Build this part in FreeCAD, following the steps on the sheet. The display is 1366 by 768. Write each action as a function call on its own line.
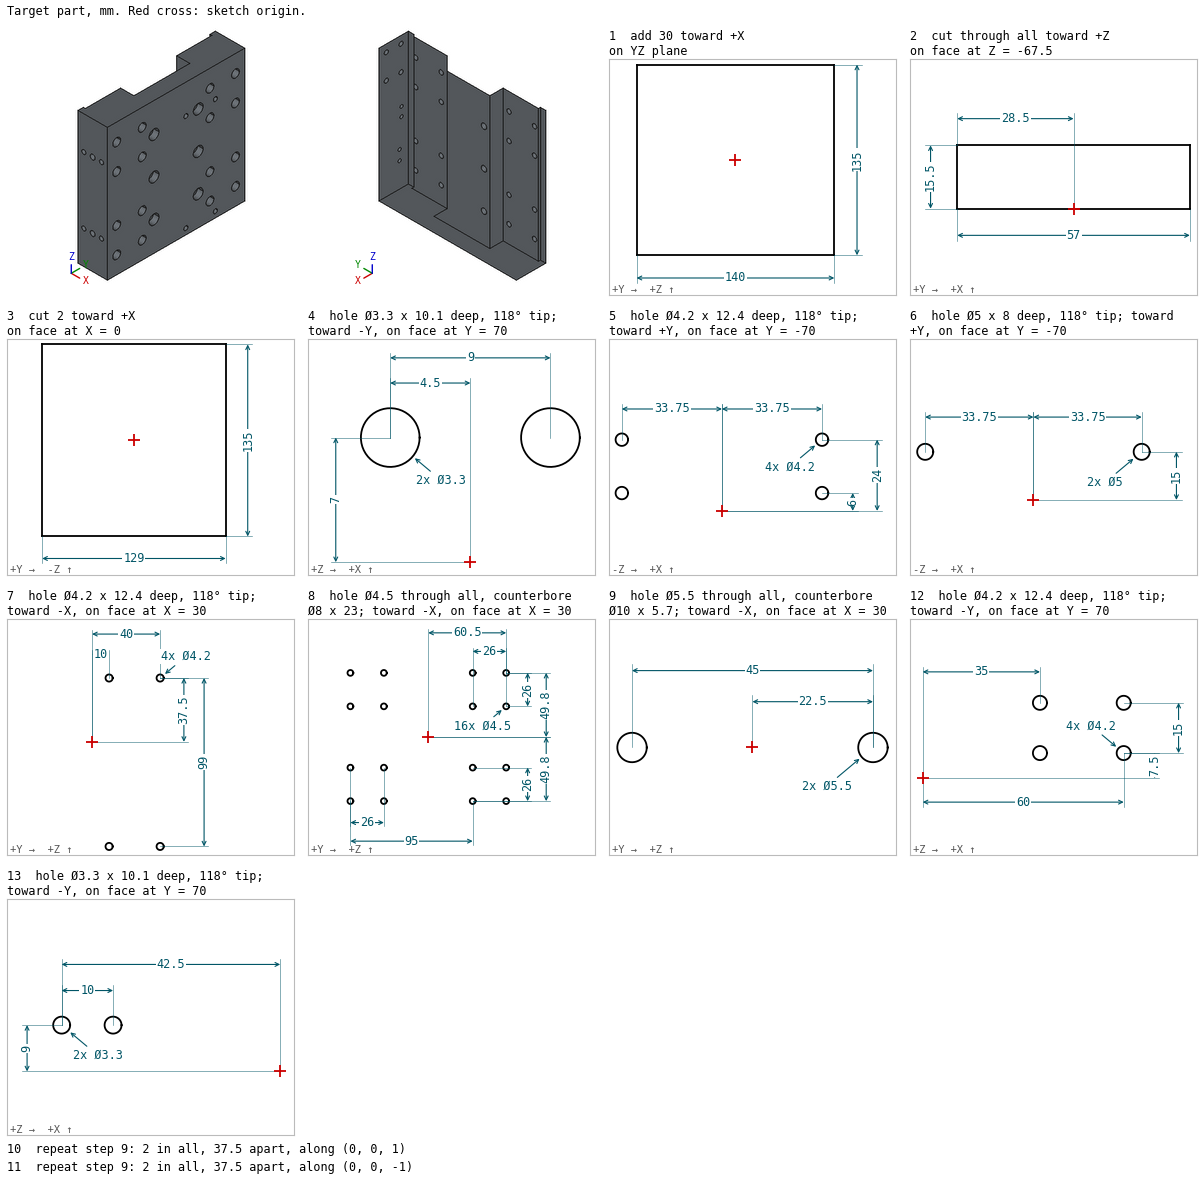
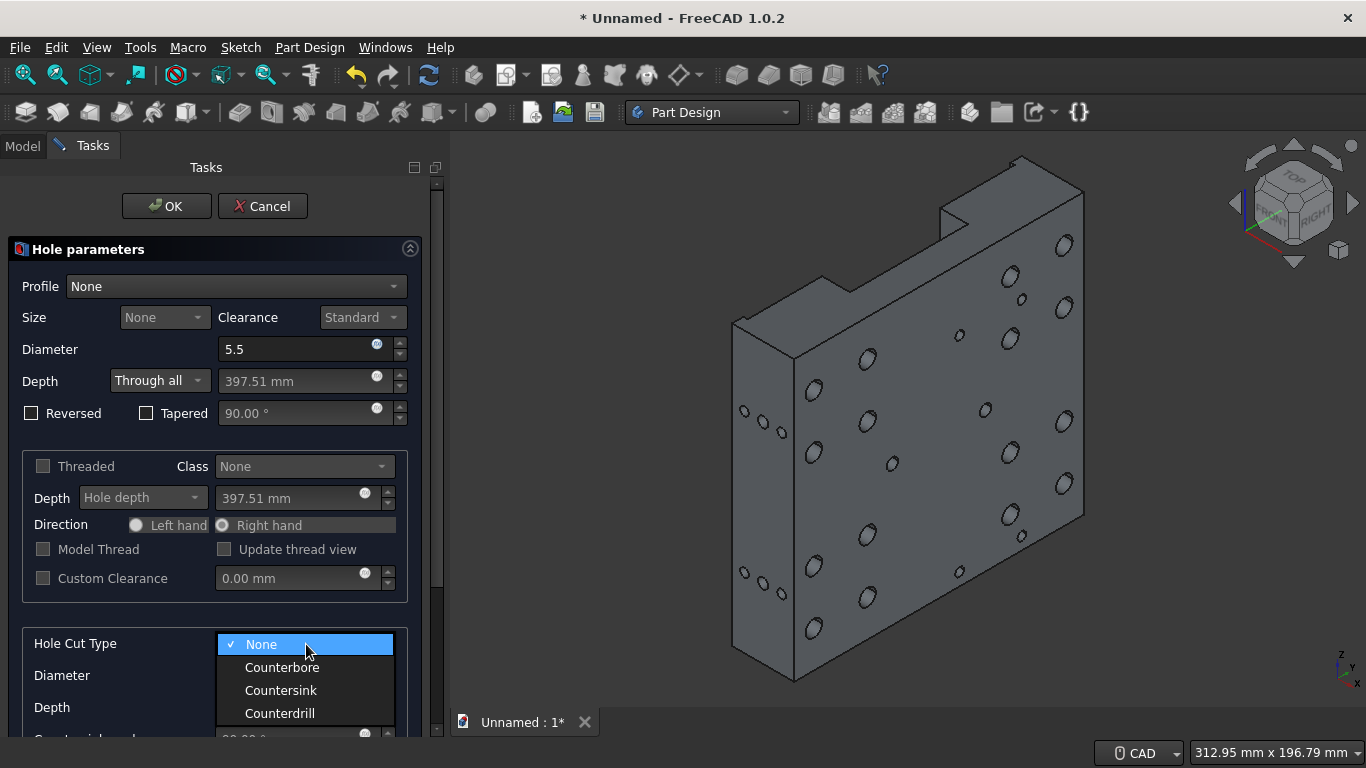
click(304, 668)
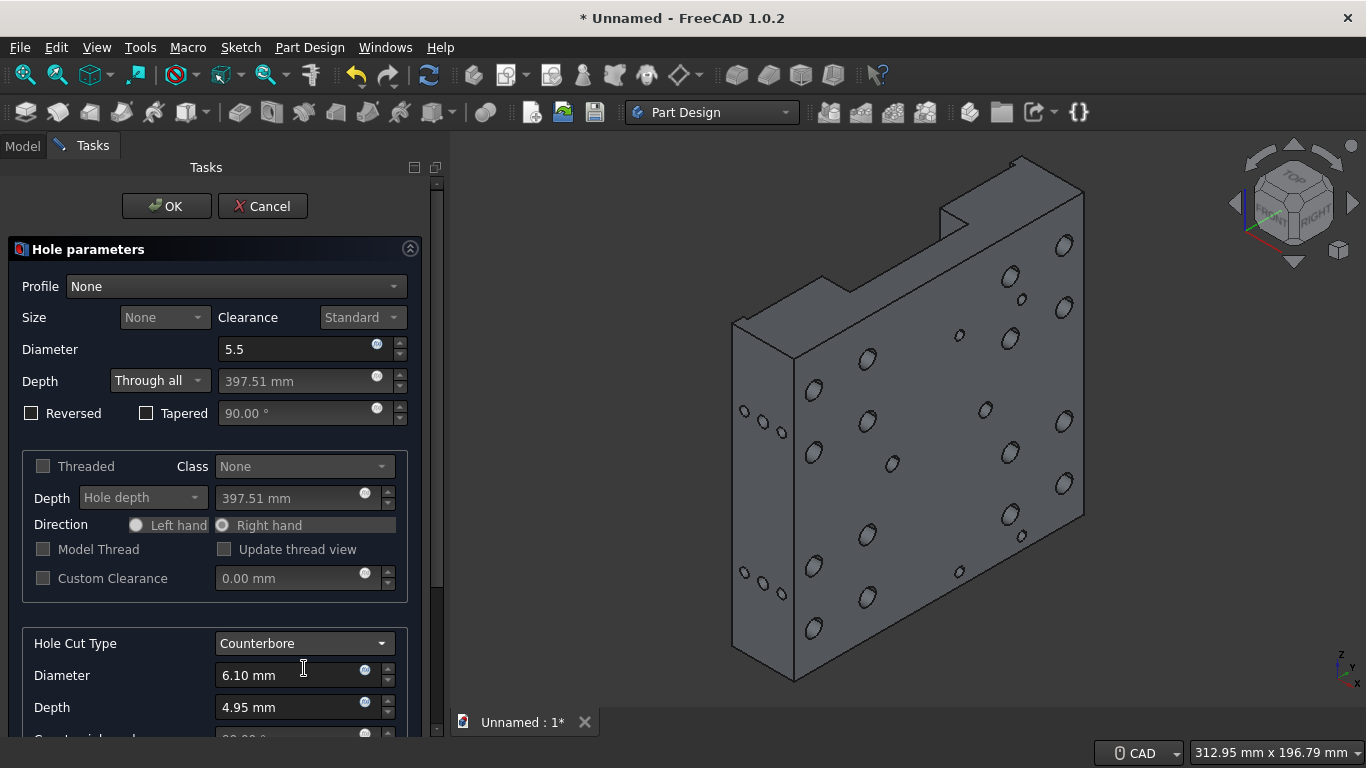
triple_click(298, 675)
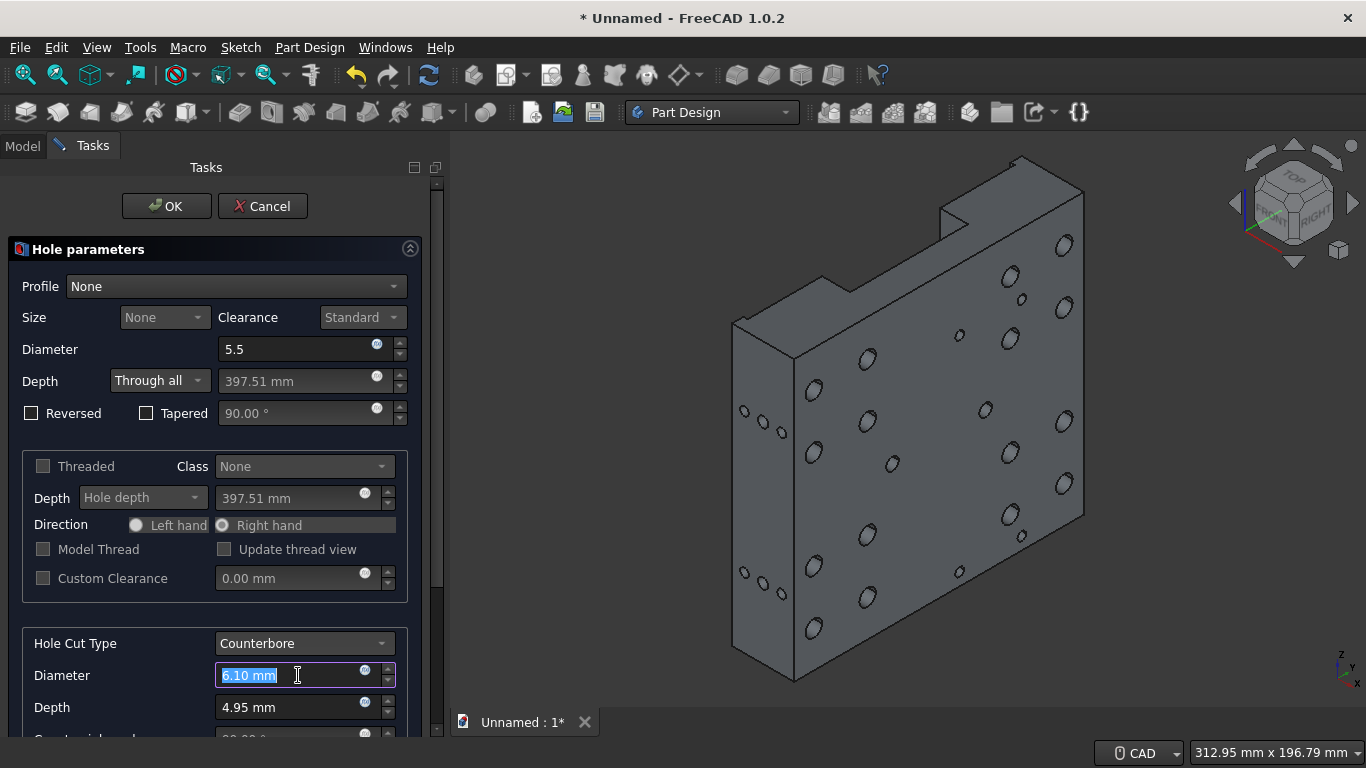
text(10)
key(Tab)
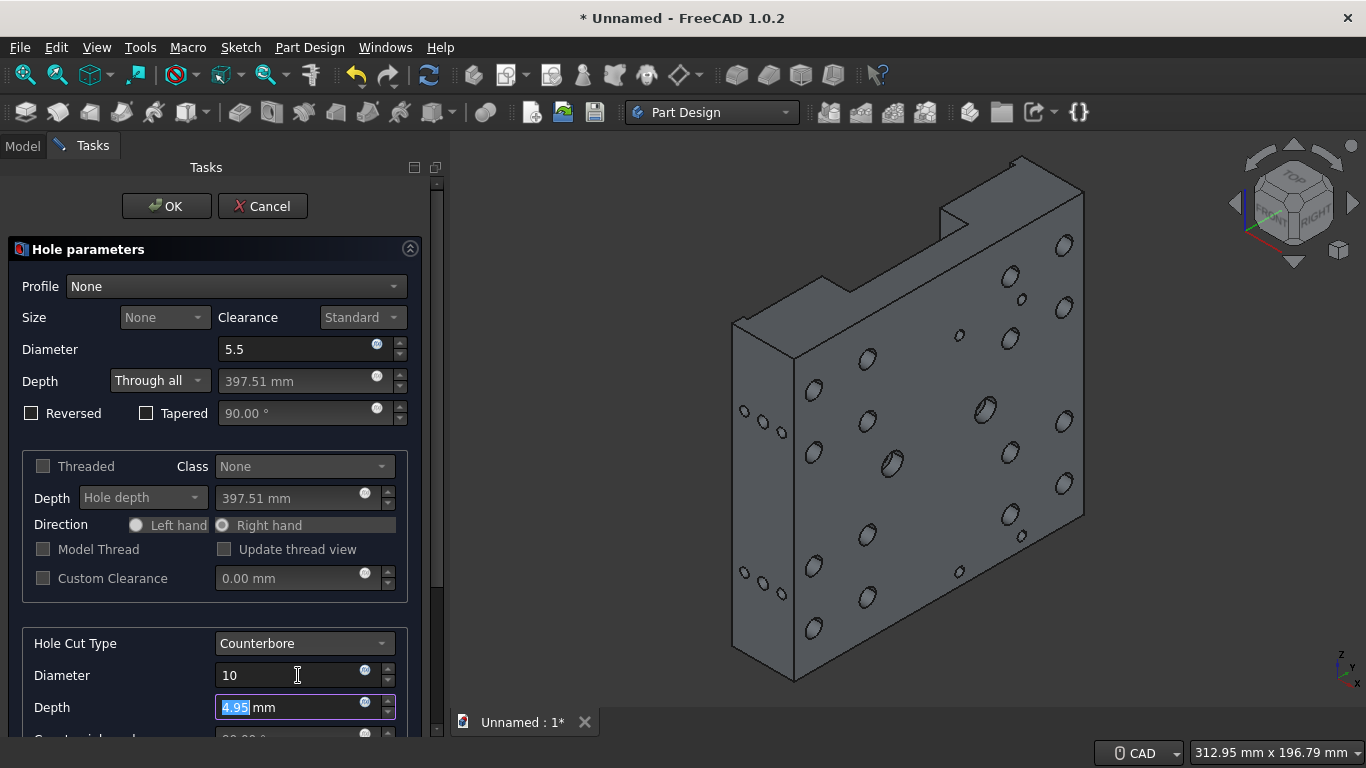
text(5.7)
key(Tab)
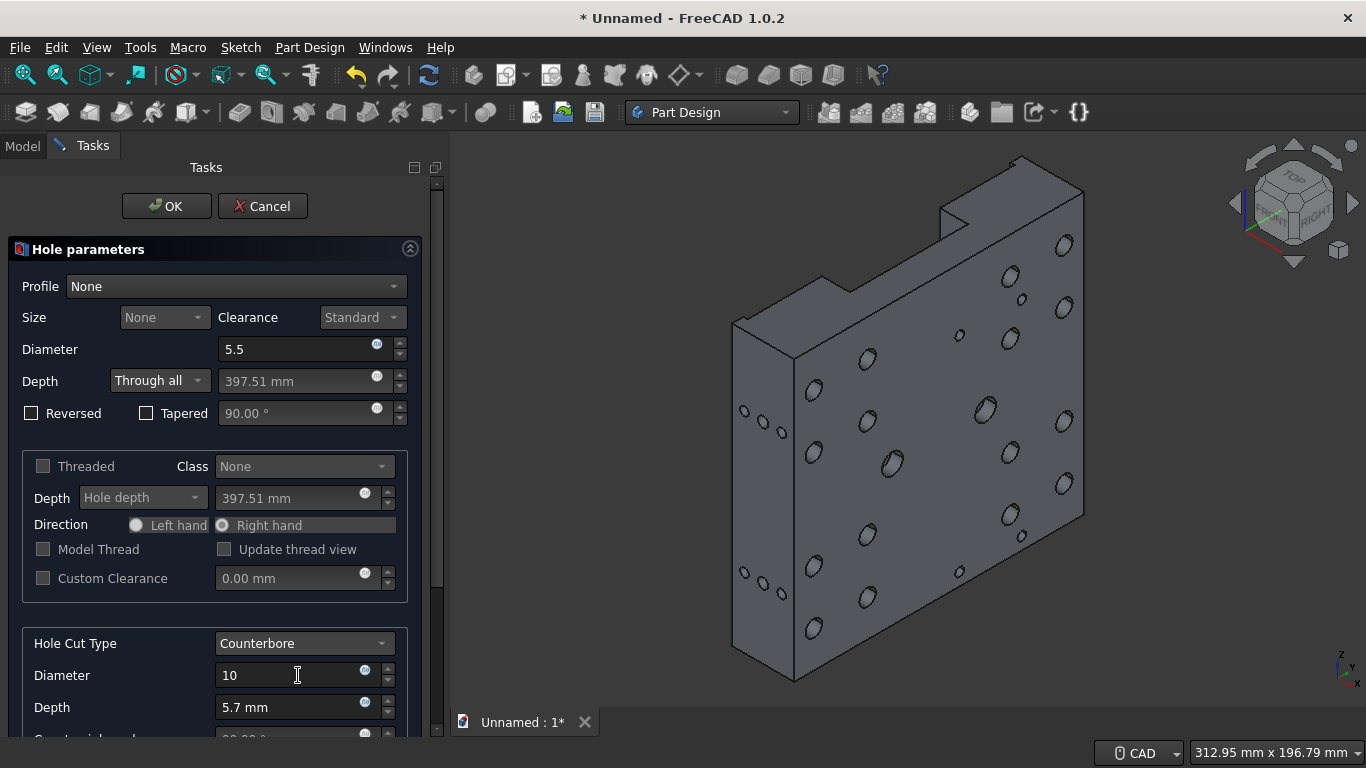
click(167, 206)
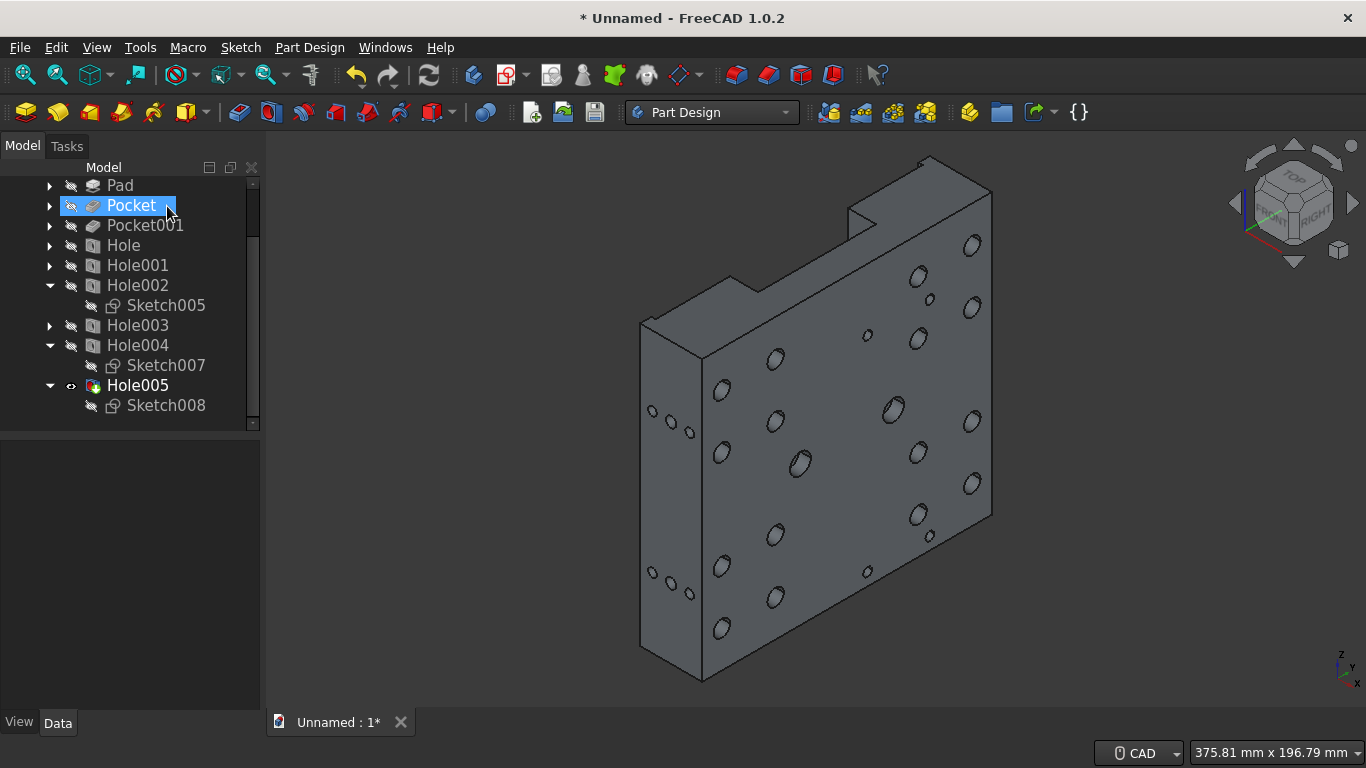
click(116, 386)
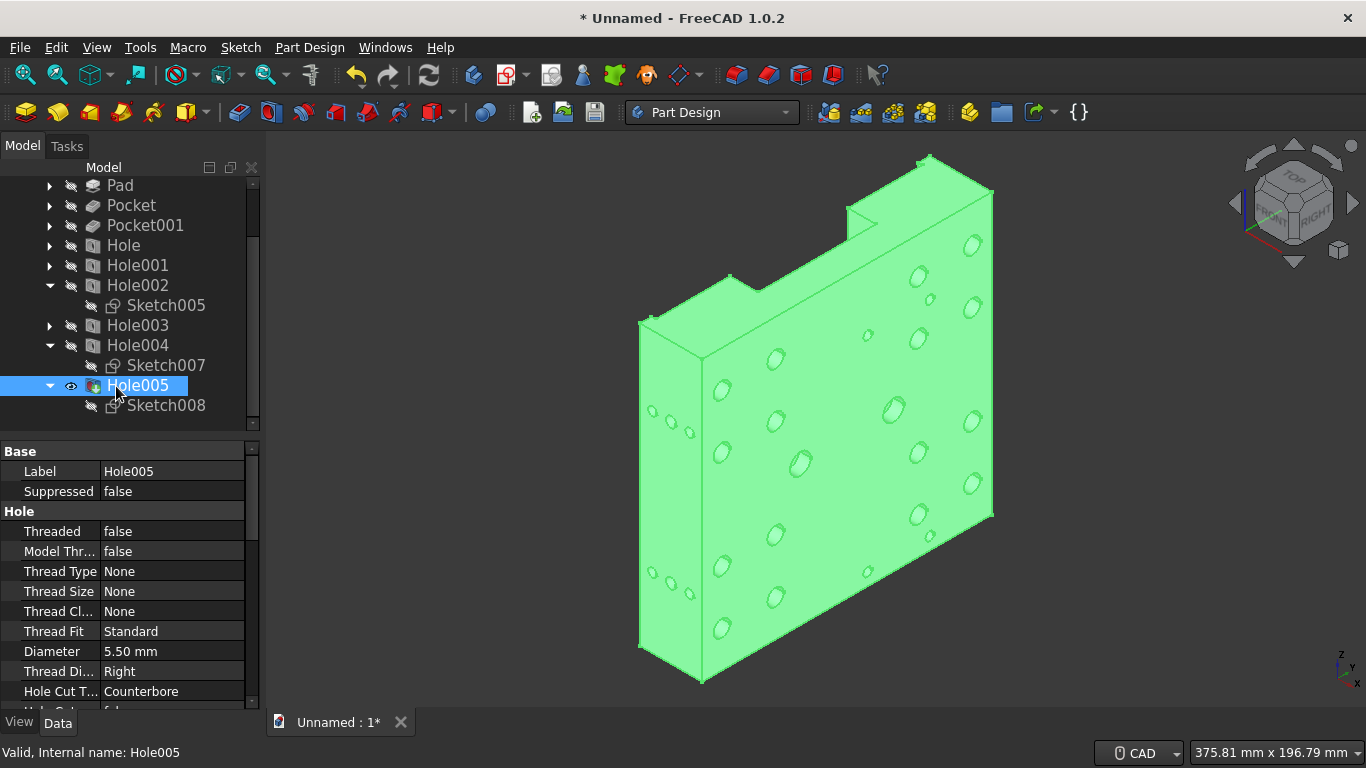
click(862, 112)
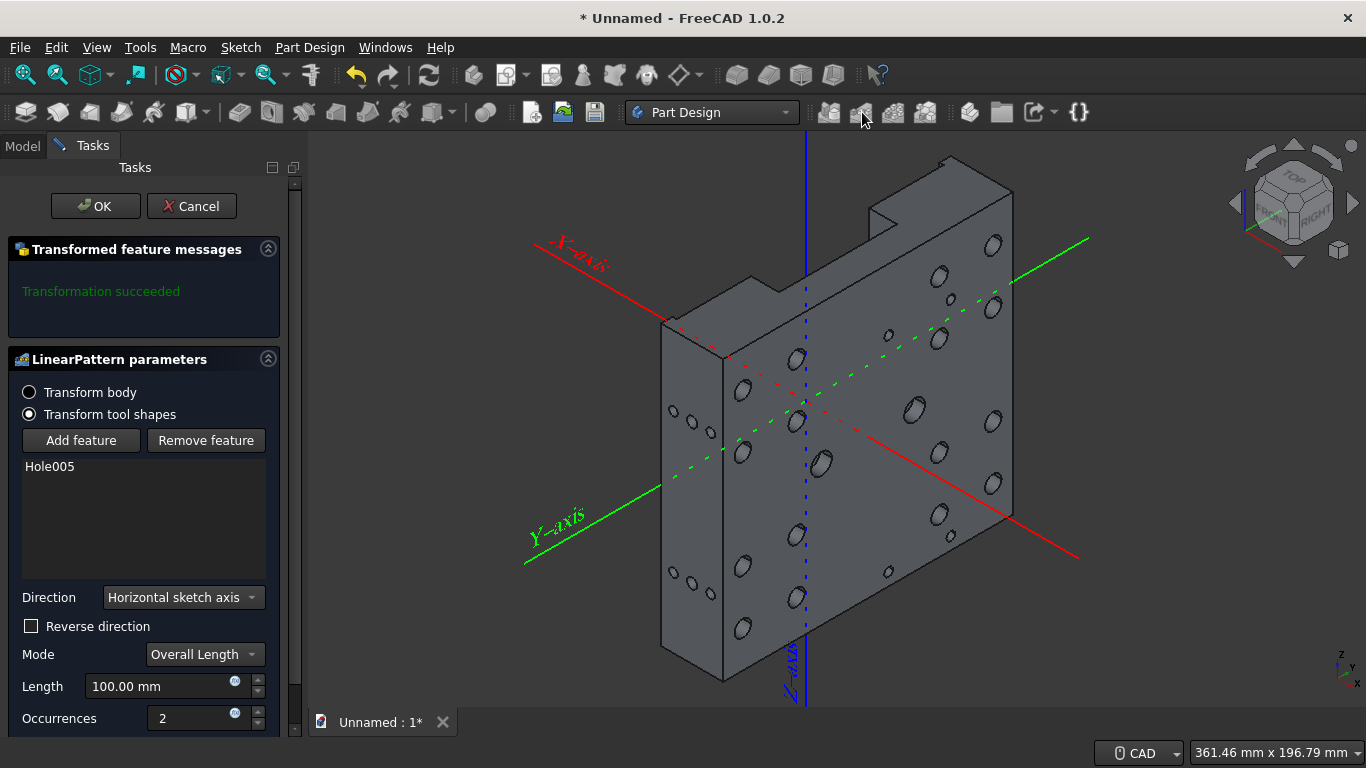
click(184, 598)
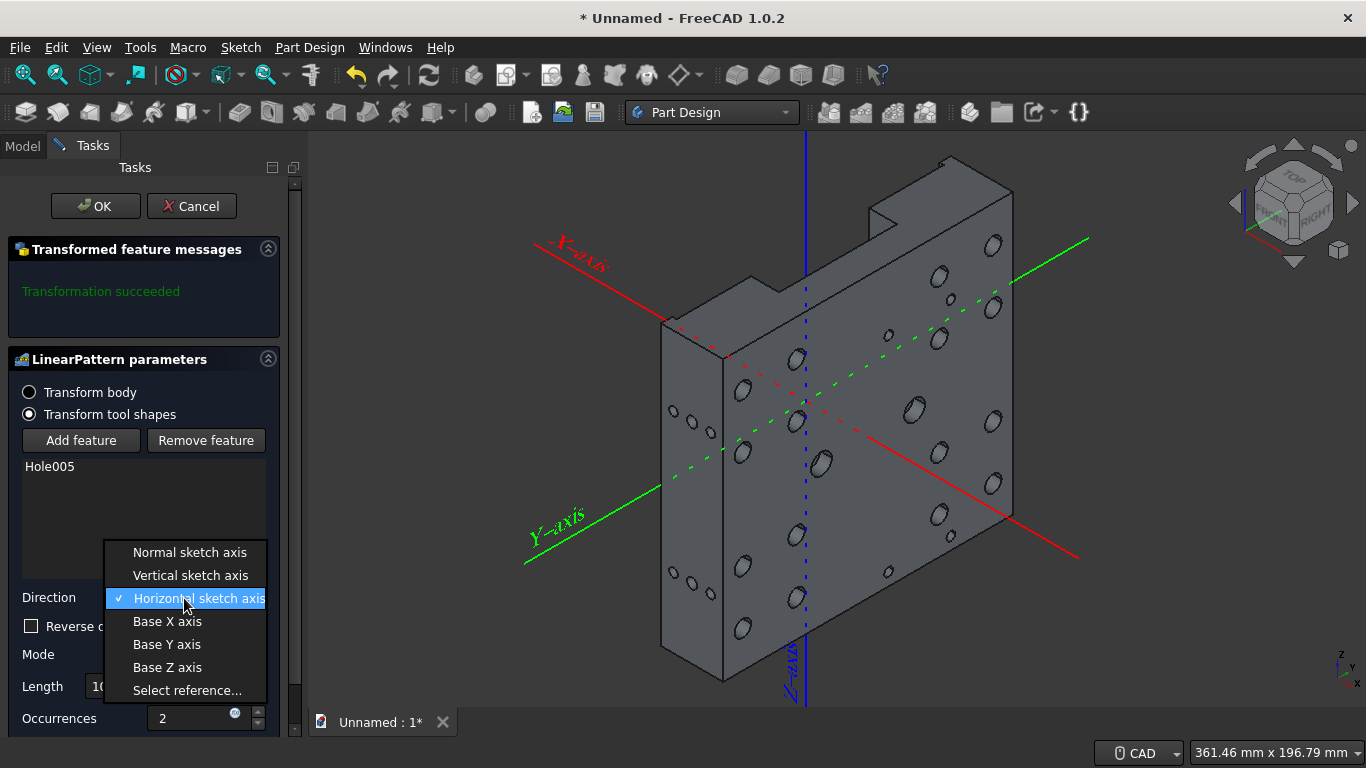
click(184, 668)